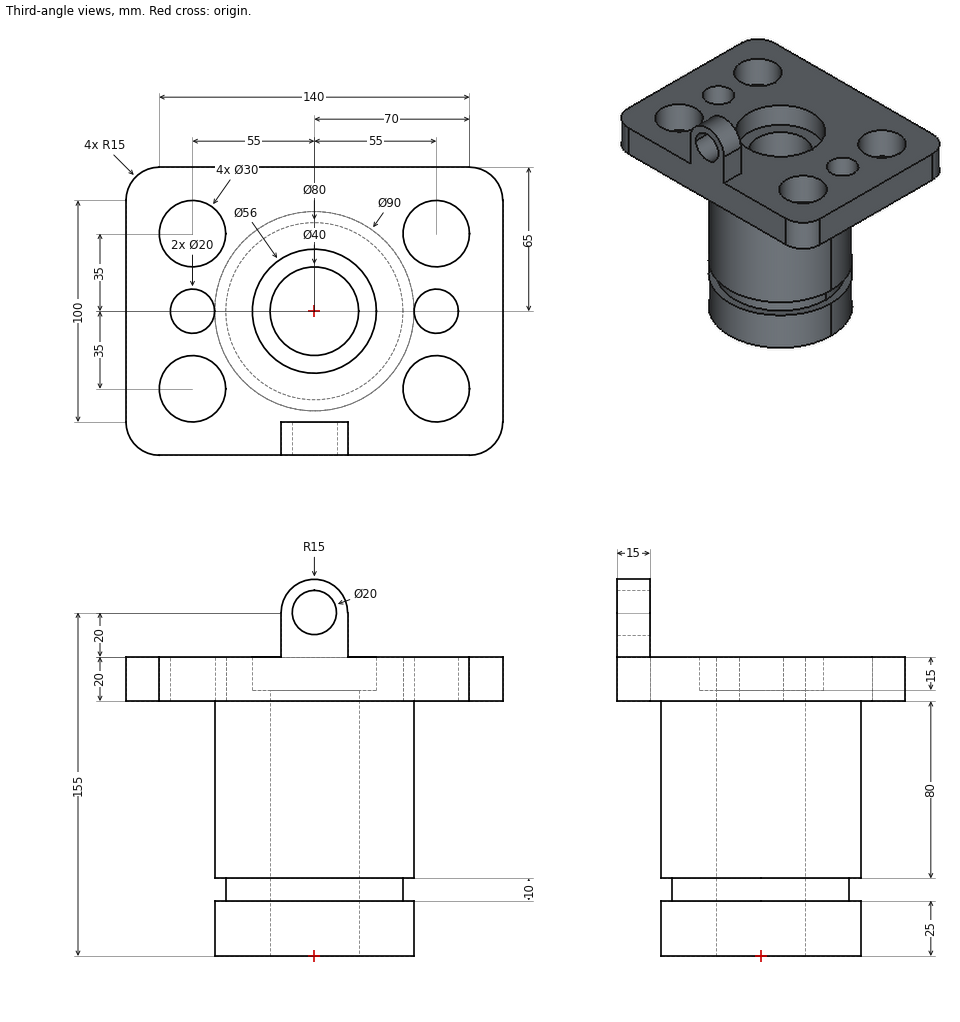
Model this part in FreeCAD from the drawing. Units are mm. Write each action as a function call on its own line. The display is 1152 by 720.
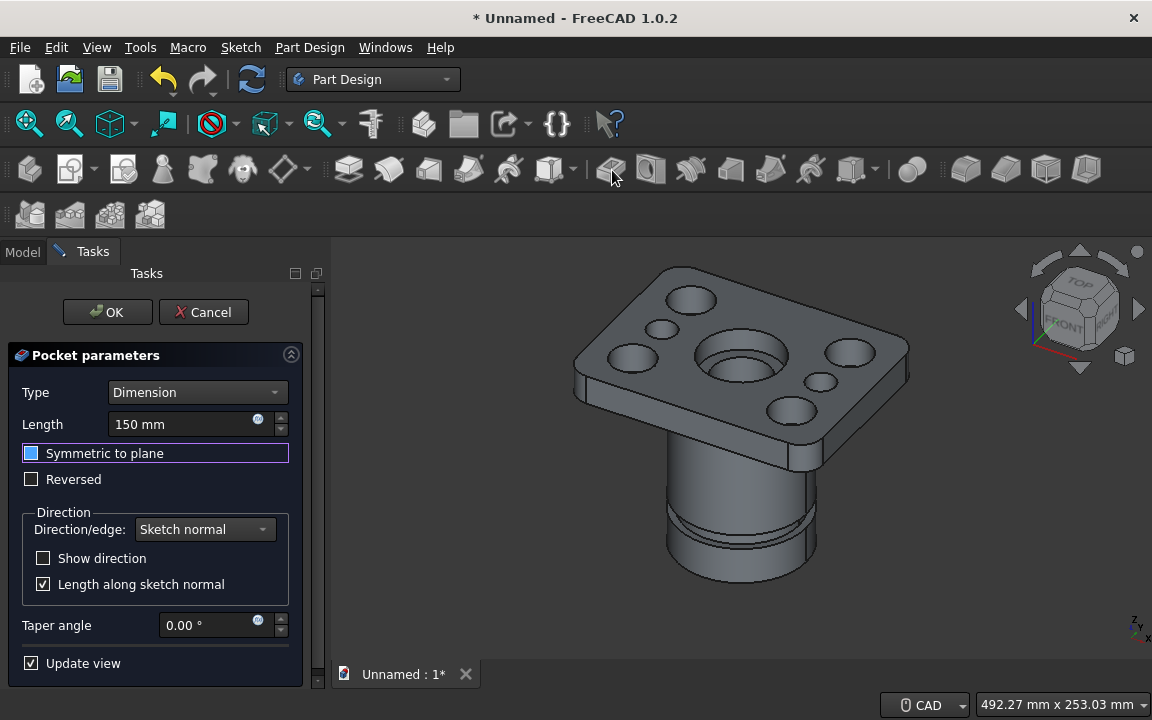
click(108, 312)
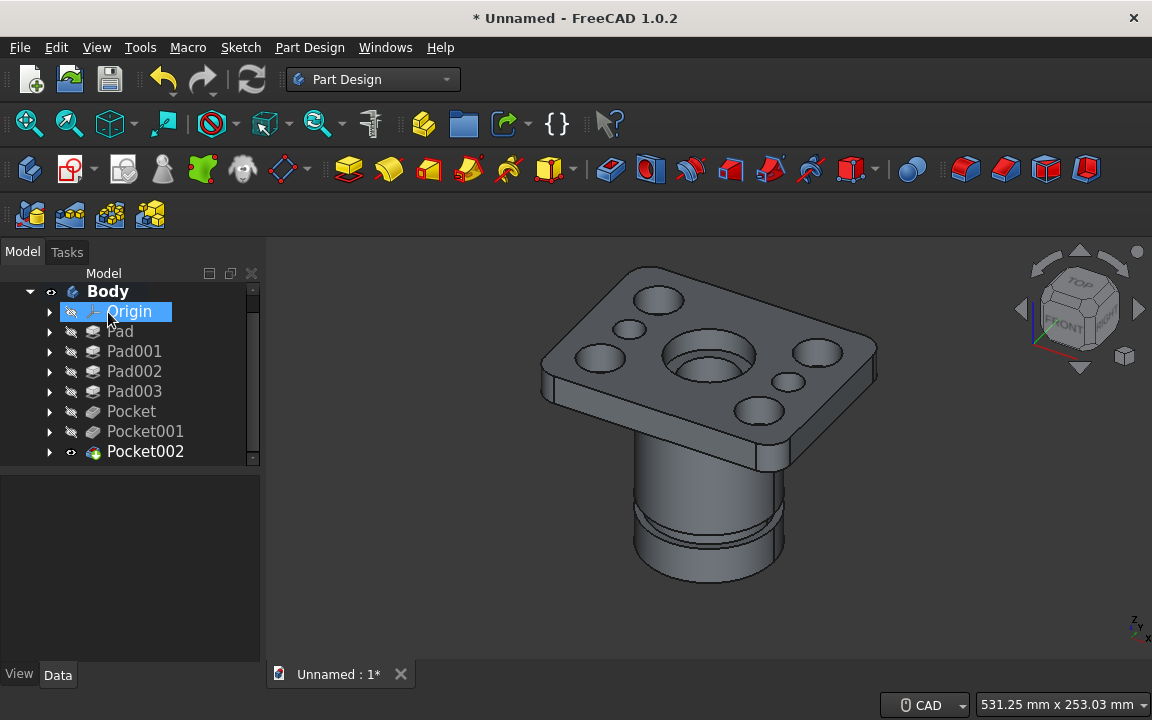
click(713, 441)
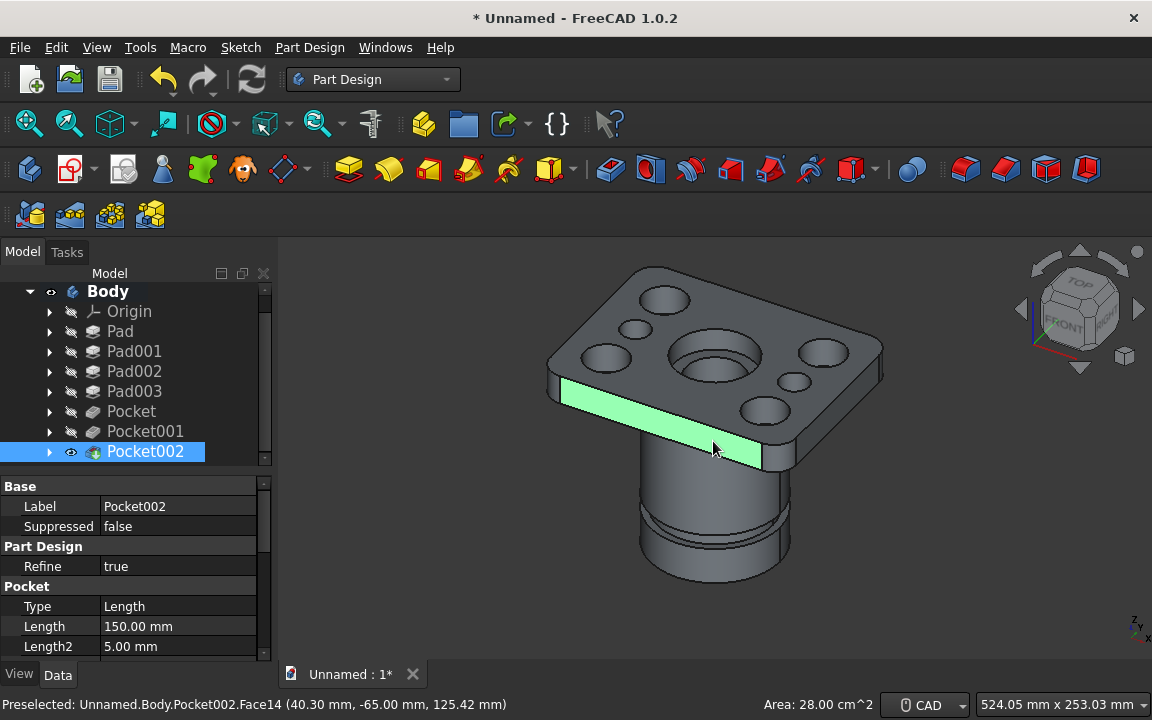
click(70, 170)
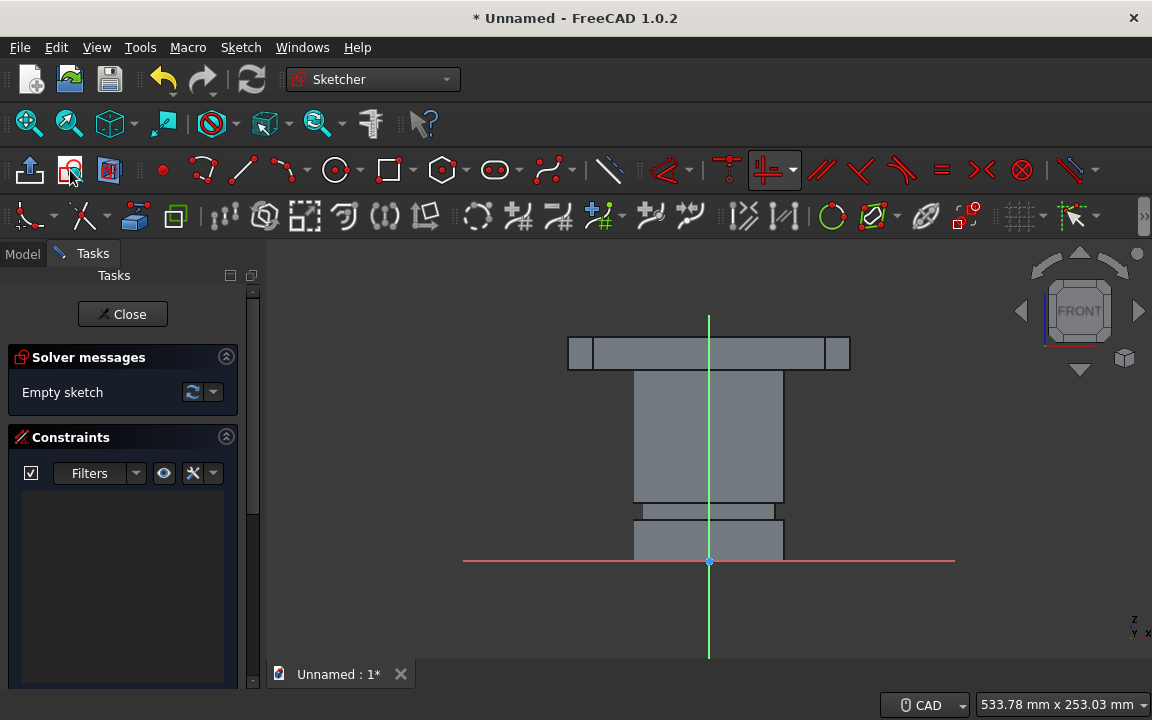
scroll(731, 267, up, 7)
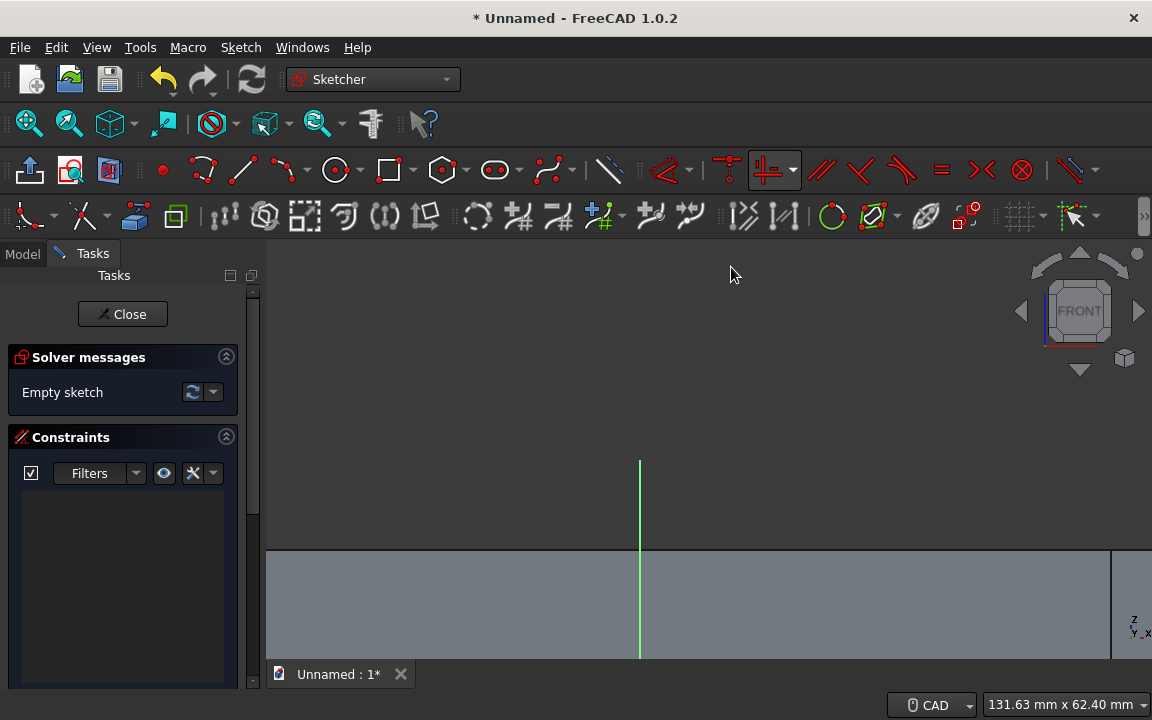
click(204, 170)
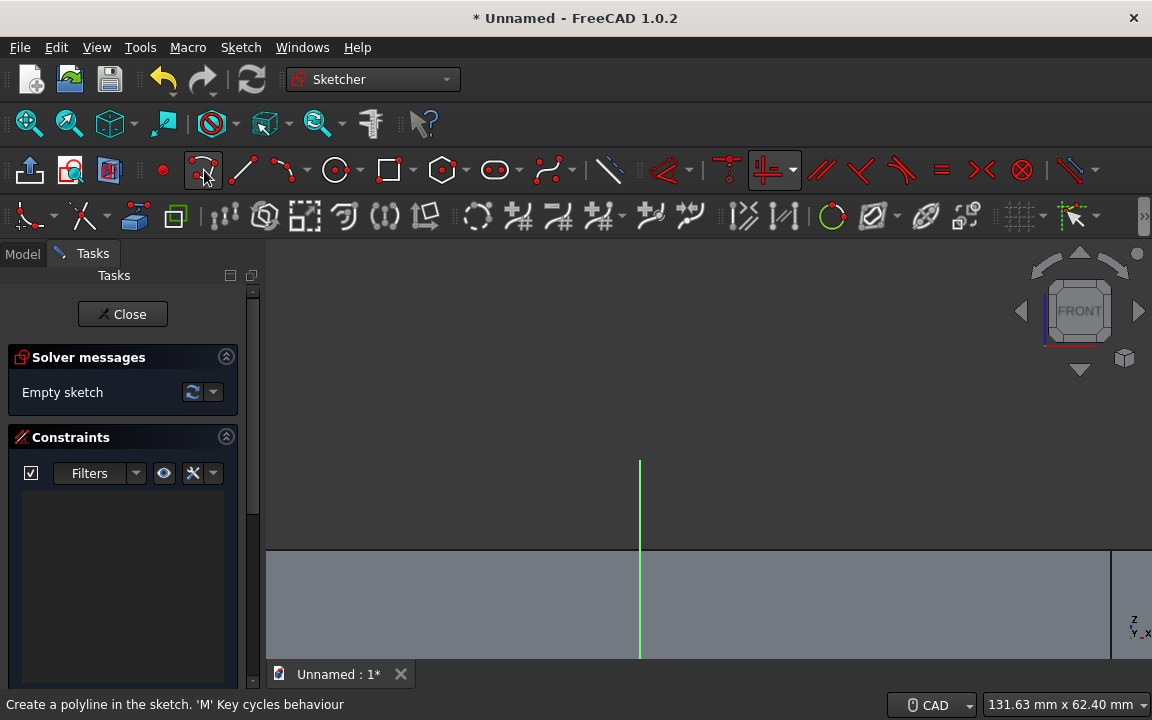
click(539, 416)
click(539, 550)
click(741, 550)
click(741, 416)
right_click(741, 416)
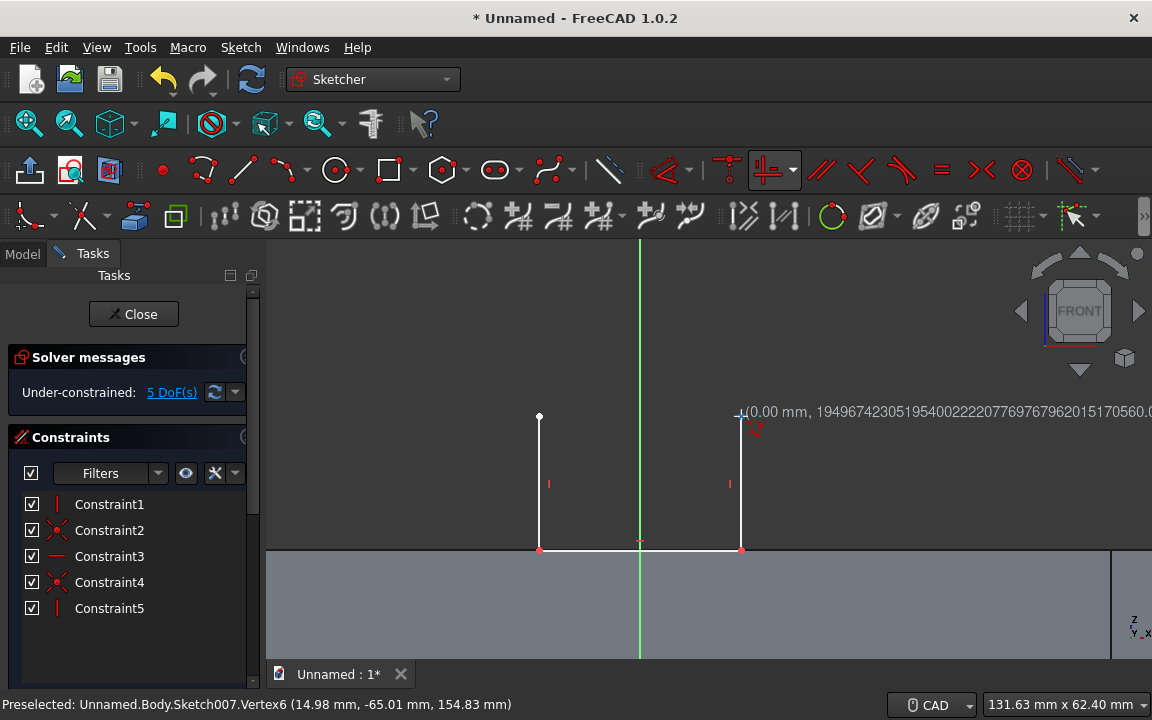
click(284, 170)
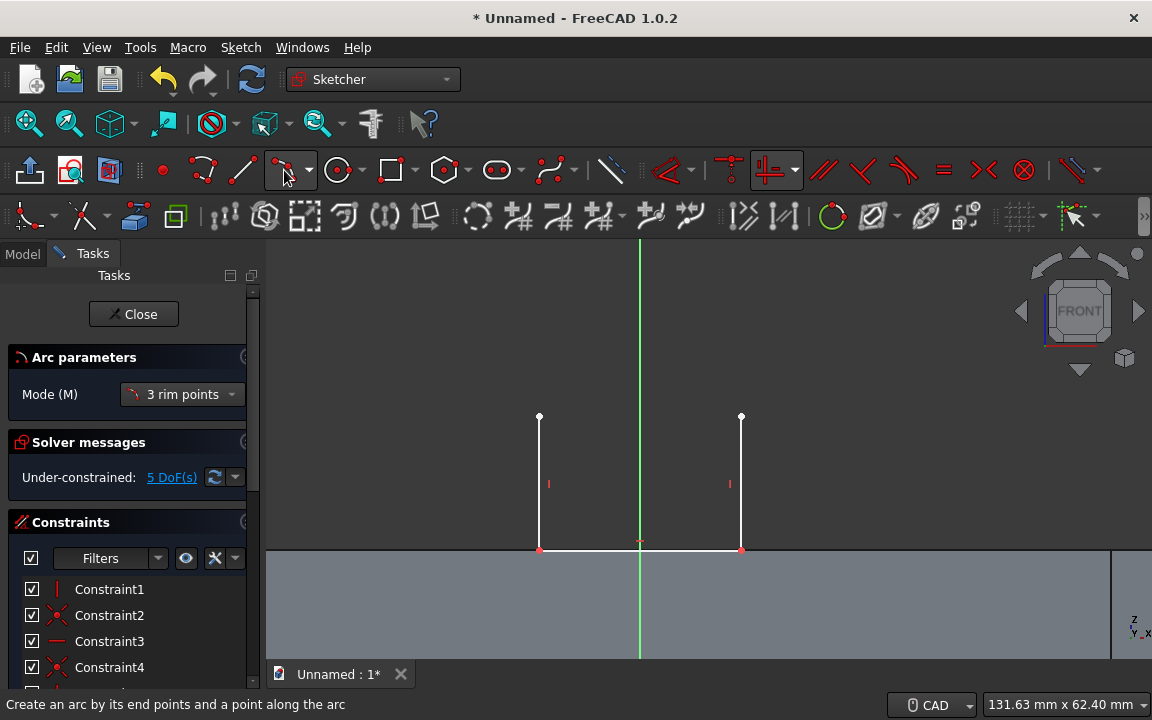
click(741, 417)
click(539, 417)
click(671, 320)
key(Escape)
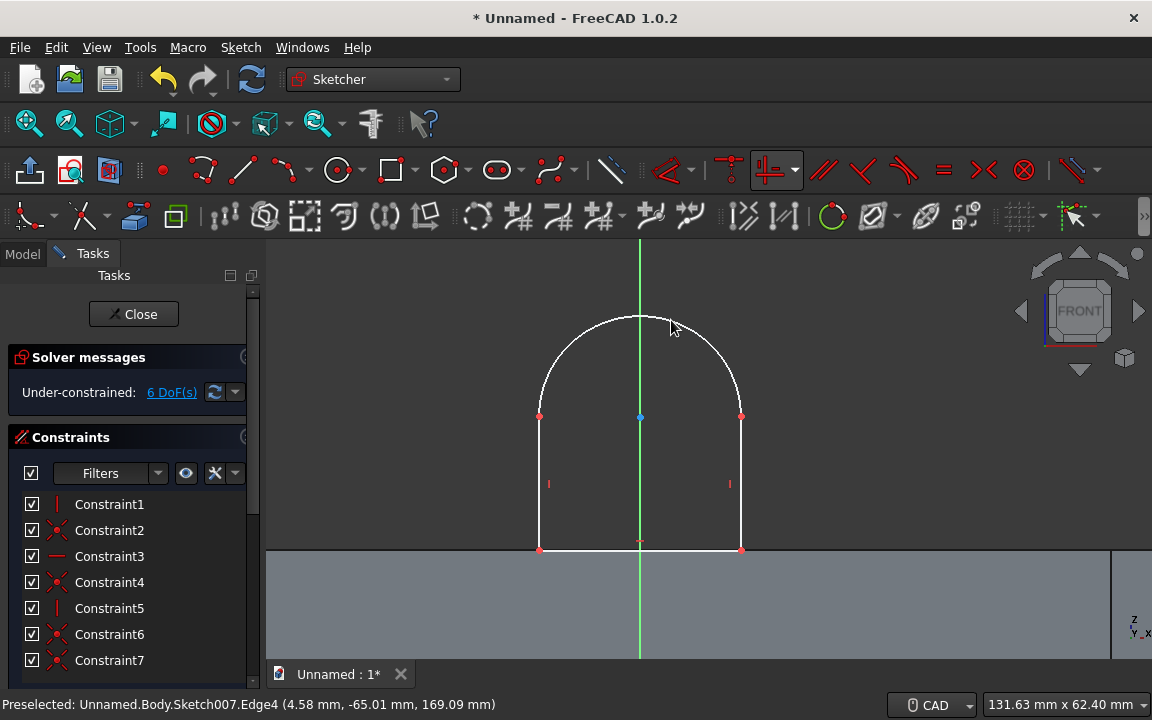
click(539, 457)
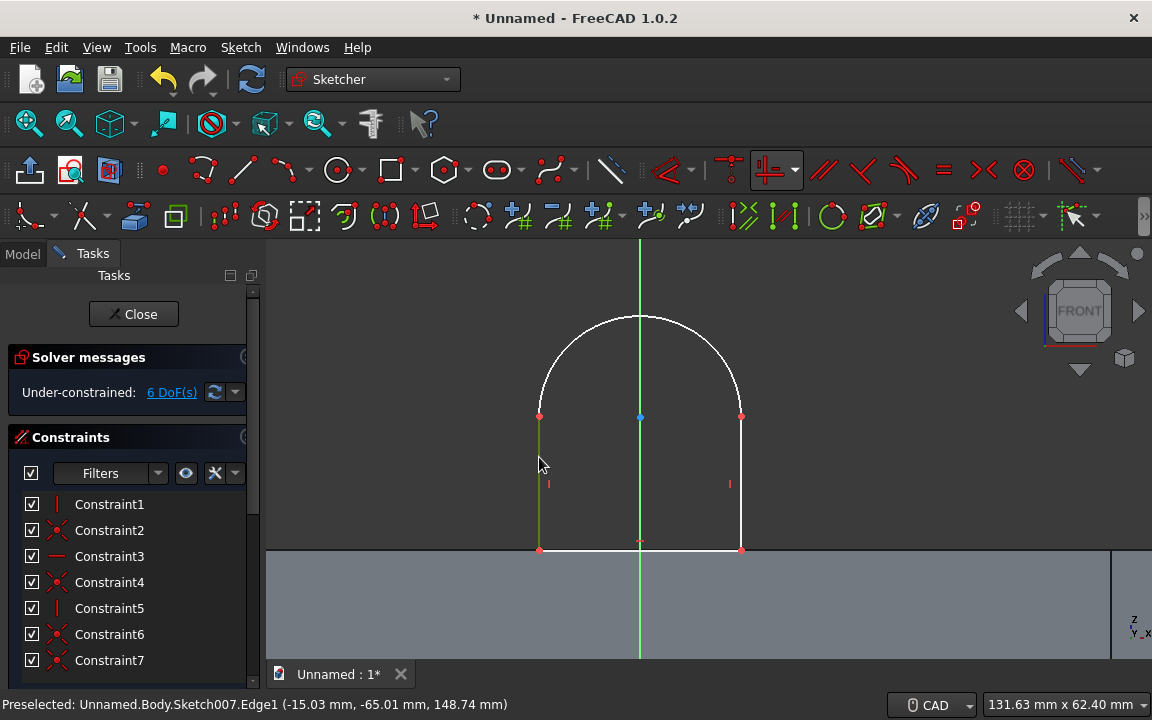
click(699, 335)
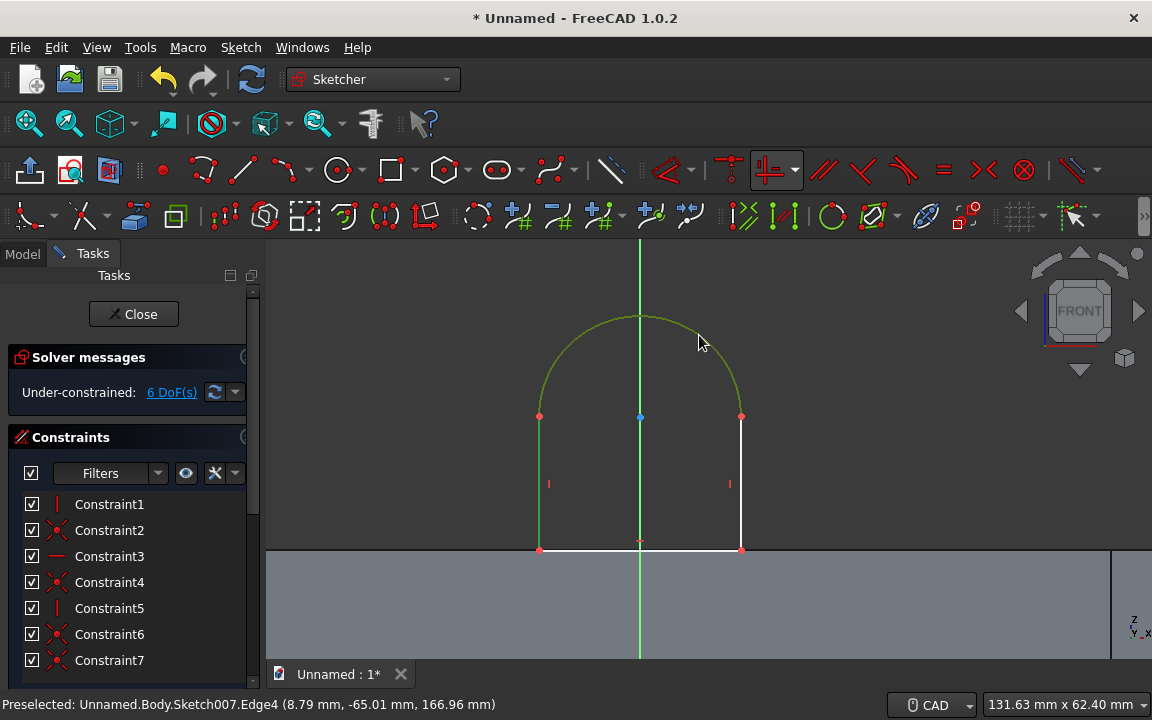
click(904, 170)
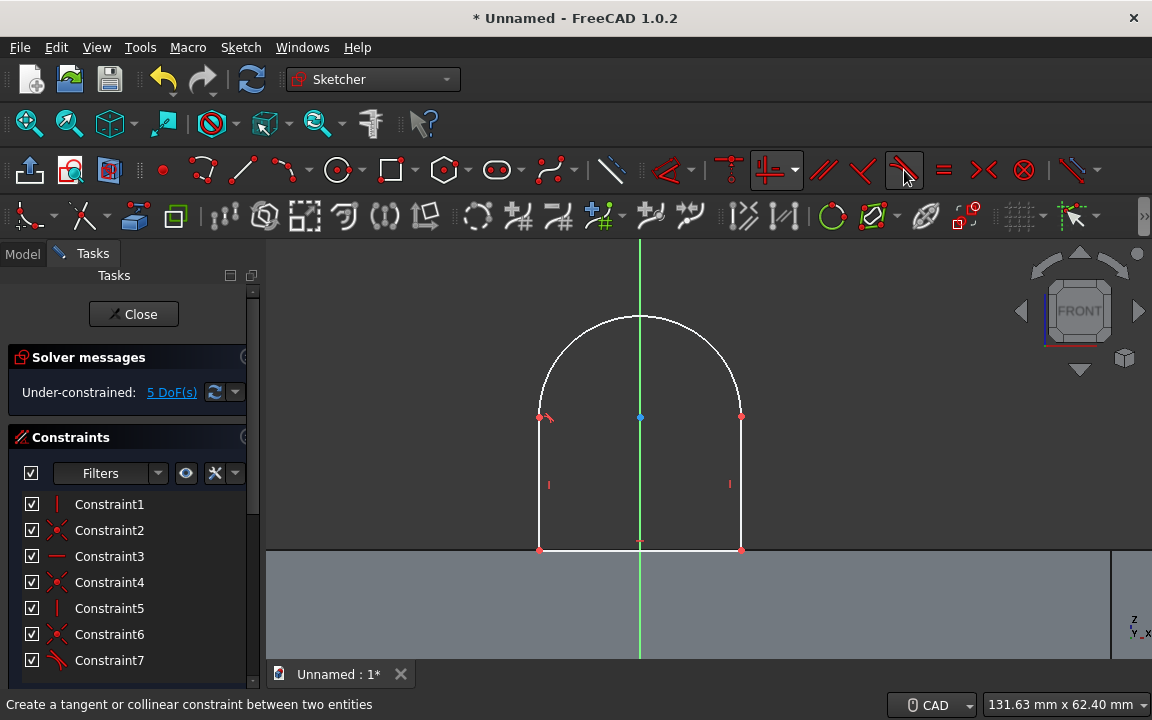
click(741, 511)